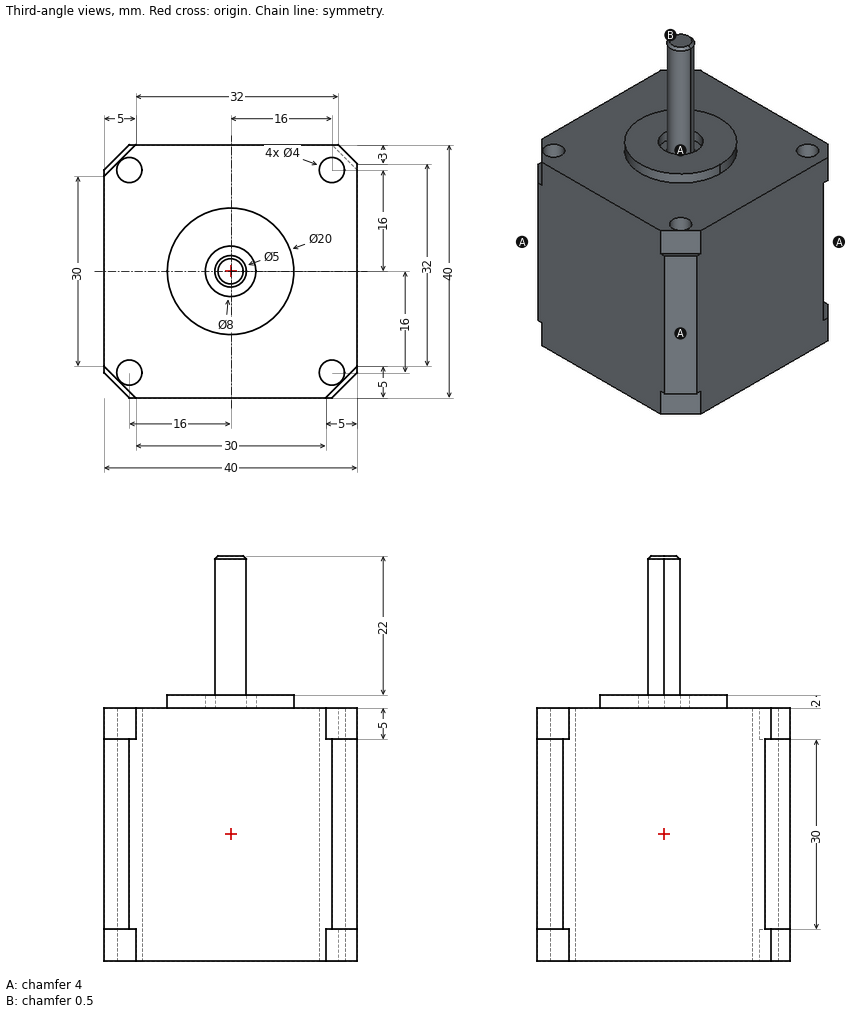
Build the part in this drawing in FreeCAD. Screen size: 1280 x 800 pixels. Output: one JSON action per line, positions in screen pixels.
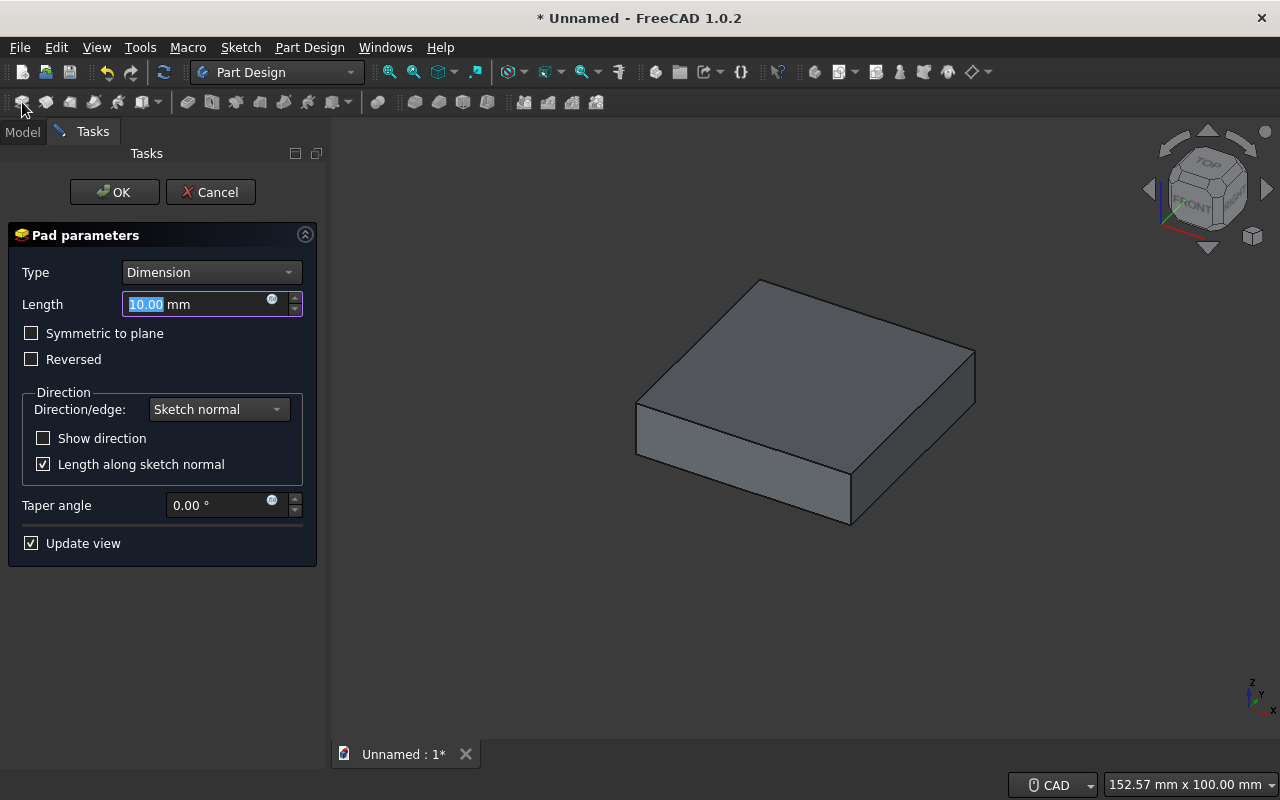
{"action": "type", "text": "30"}
{"action": "key", "text": "Tab"}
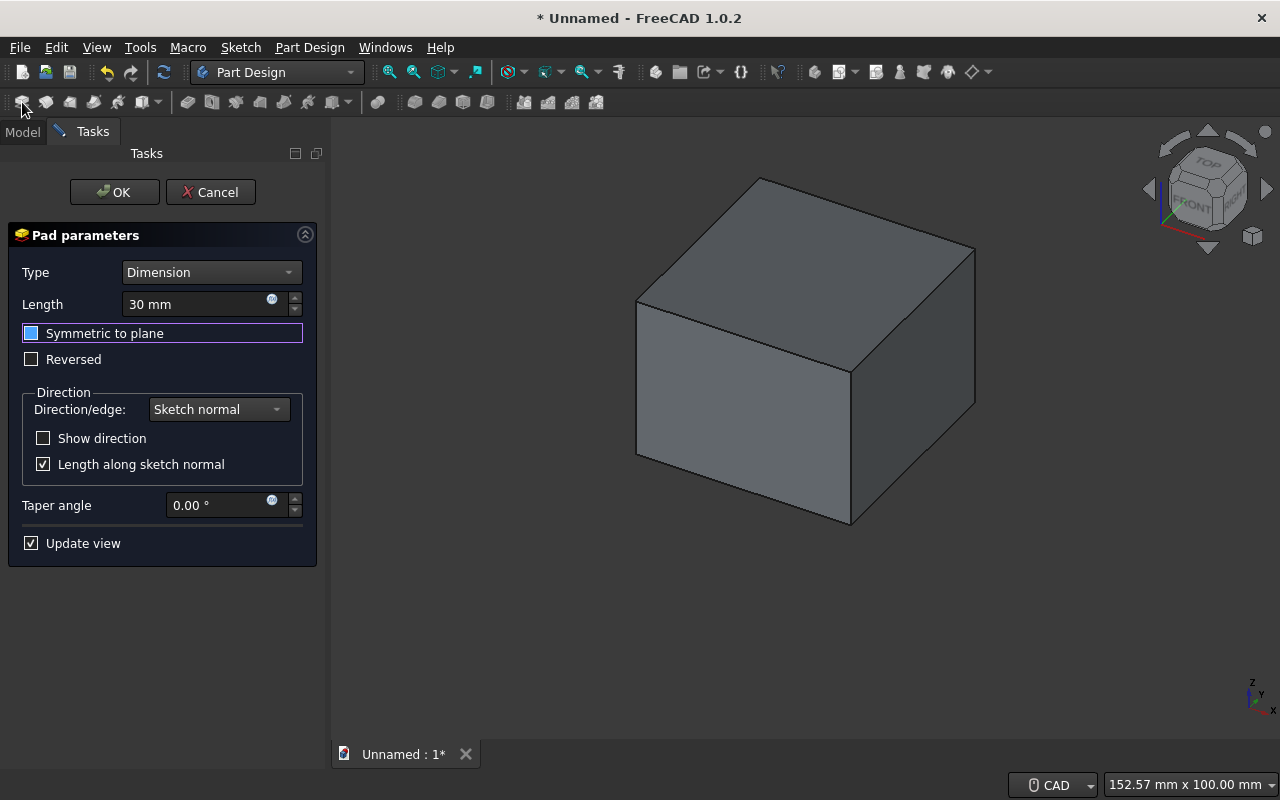
{"action": "left_click", "coordinate": [30, 333]}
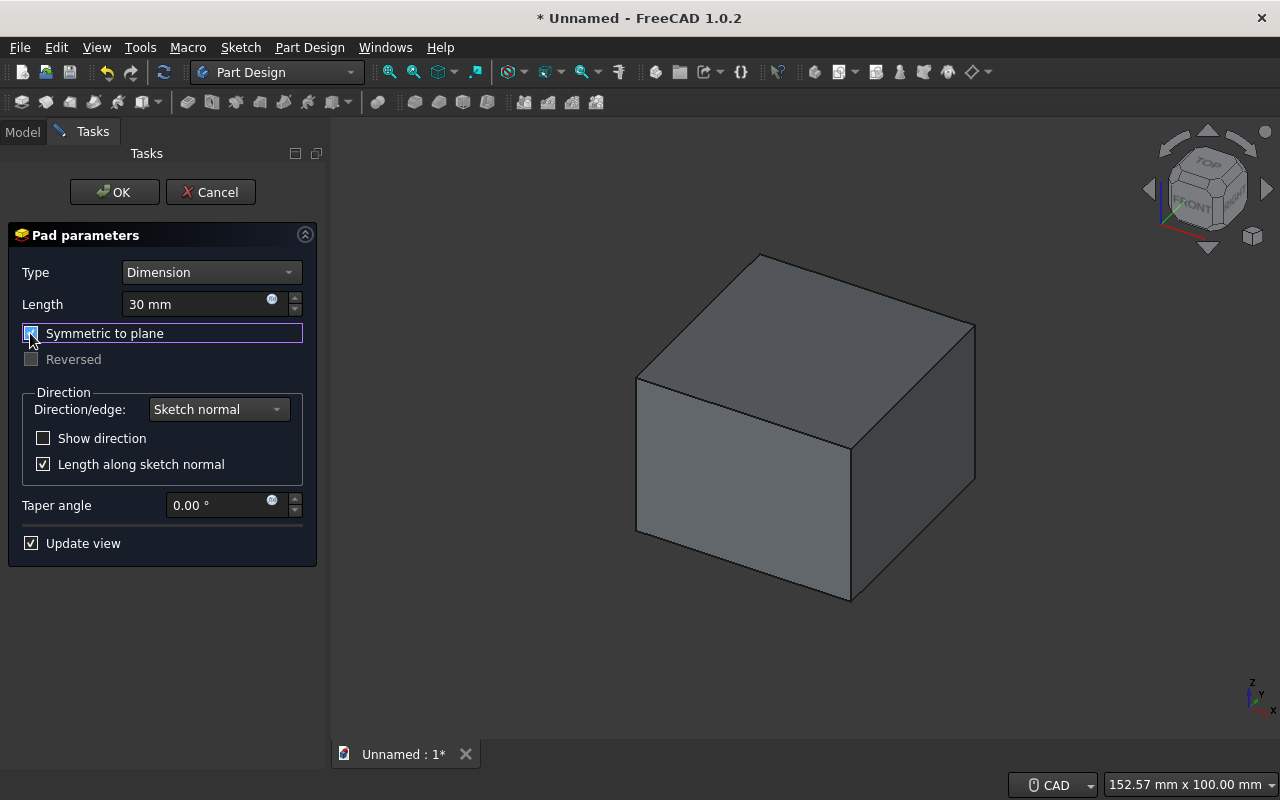
{"action": "left_click", "coordinate": [115, 192]}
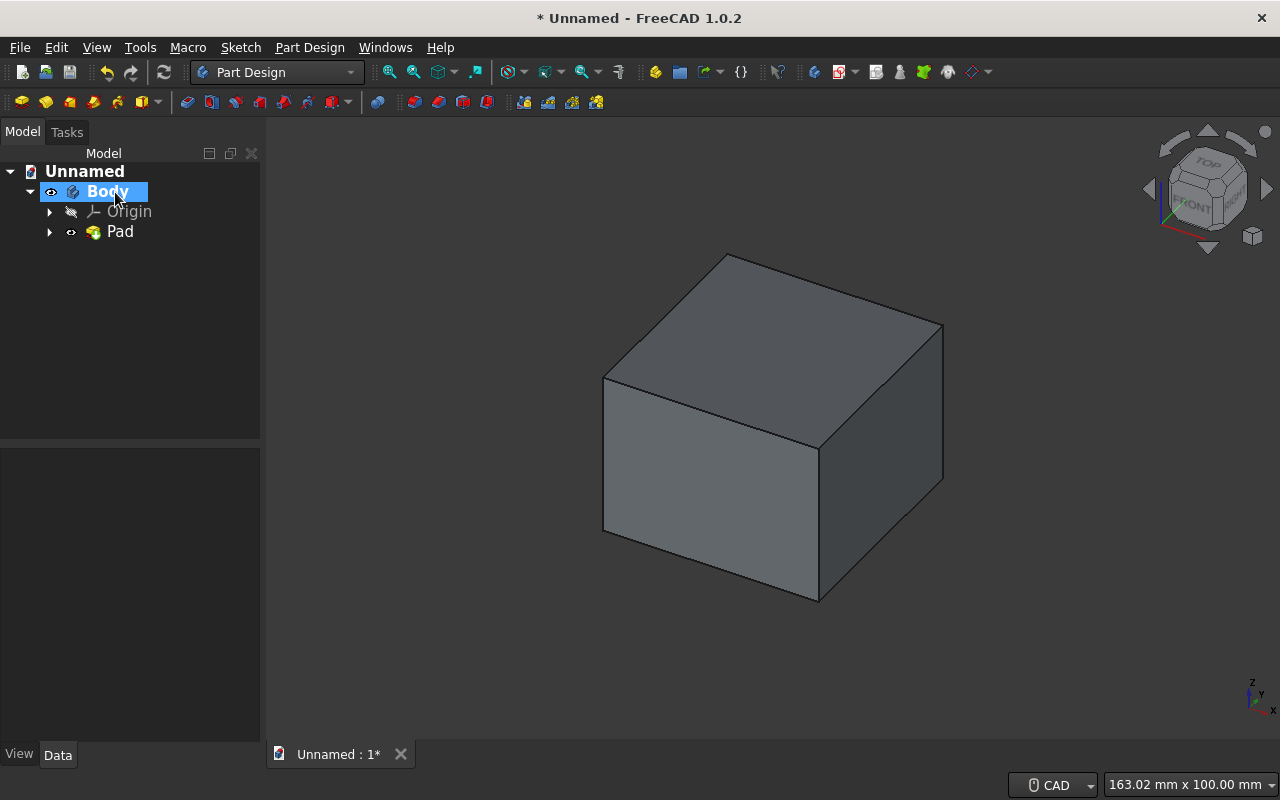
{"action": "left_click", "coordinate": [819, 524]}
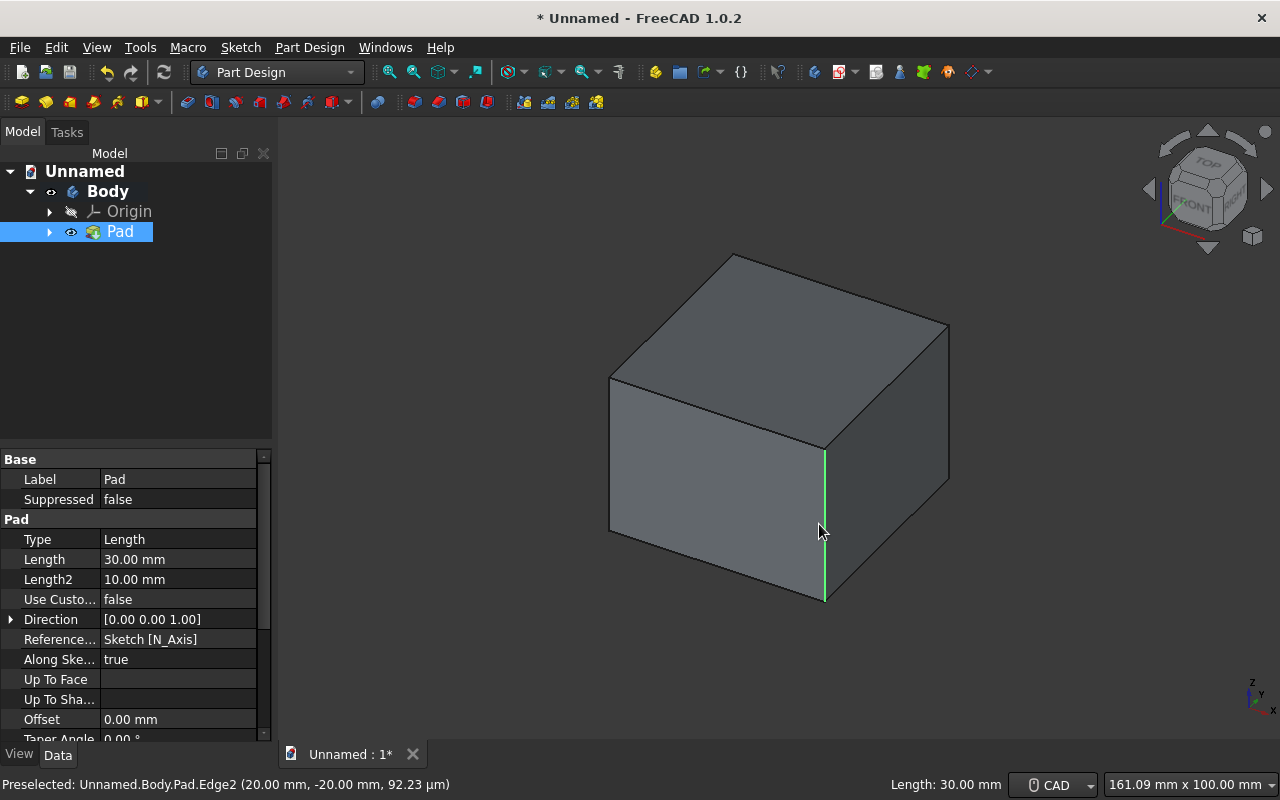
{"action": "key", "text": "0"}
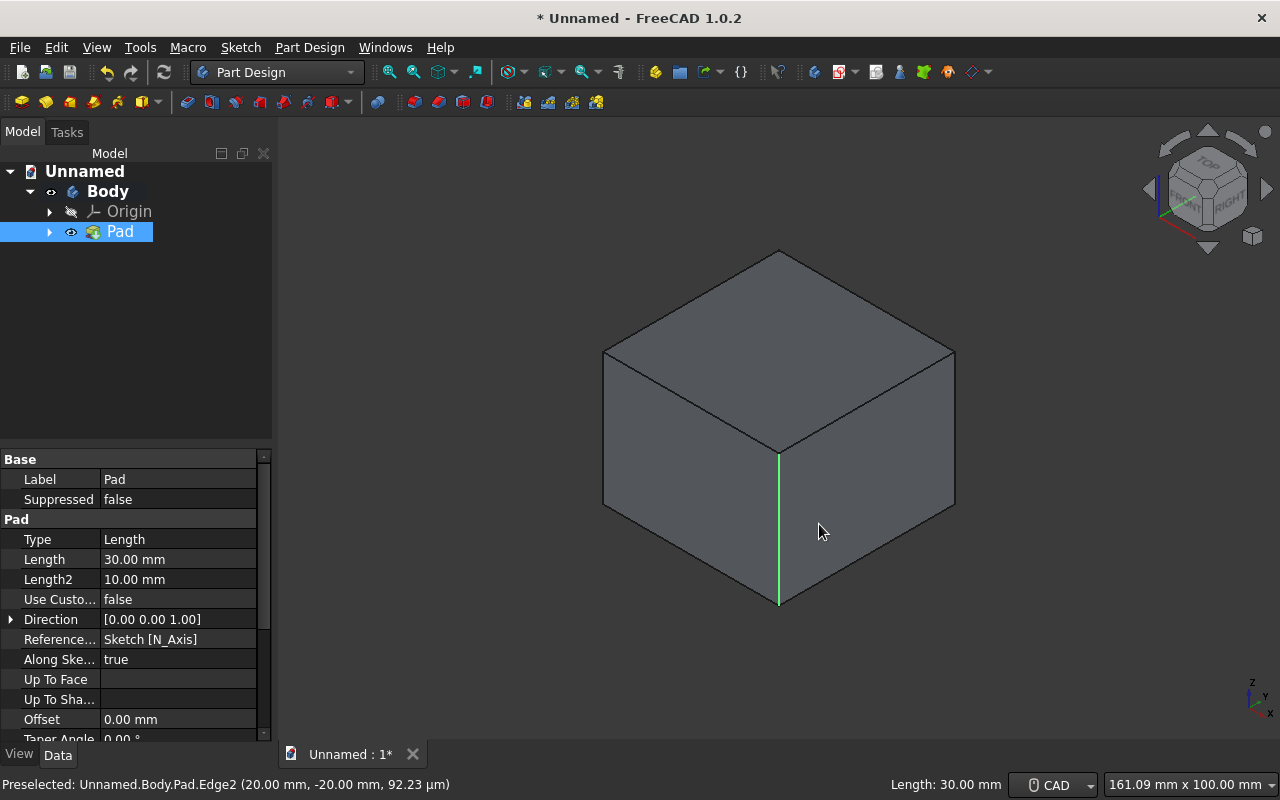
{"action": "key", "text": "2"}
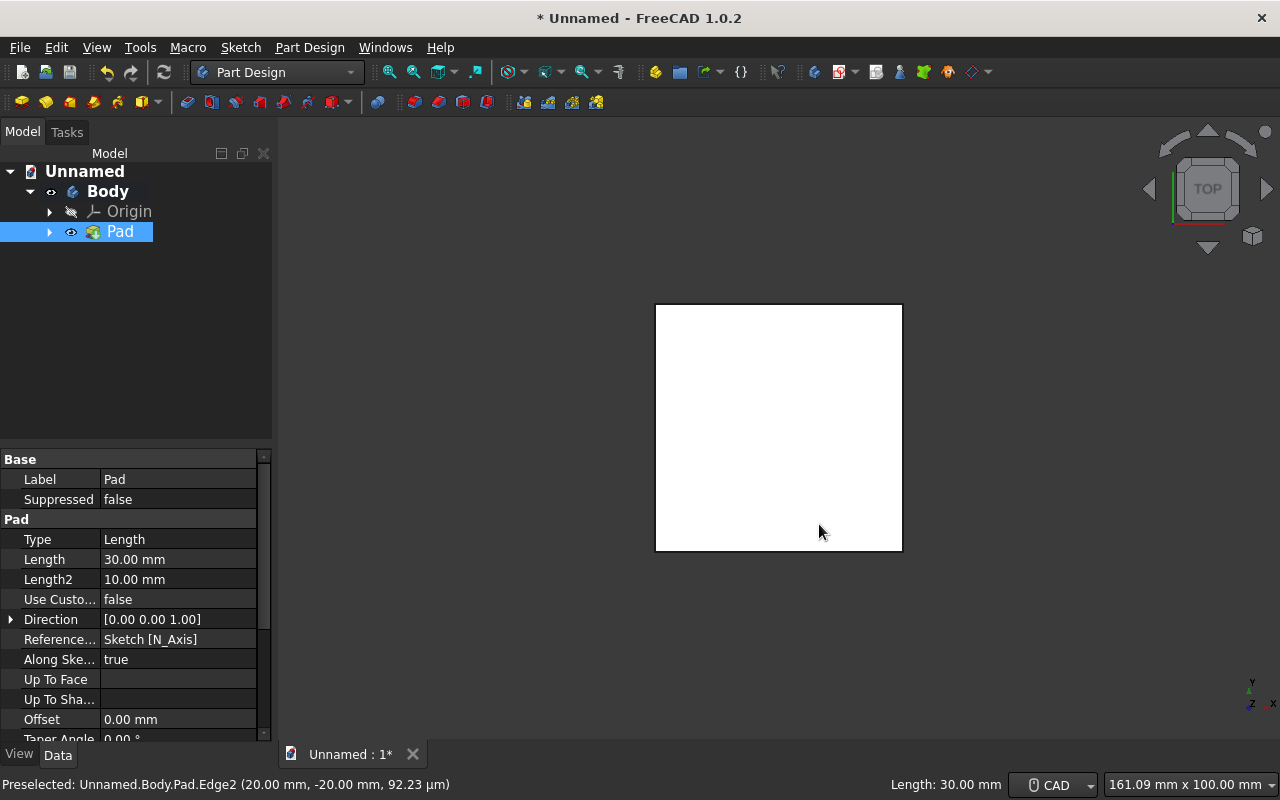
{"action": "left_click", "coordinate": [390, 72]}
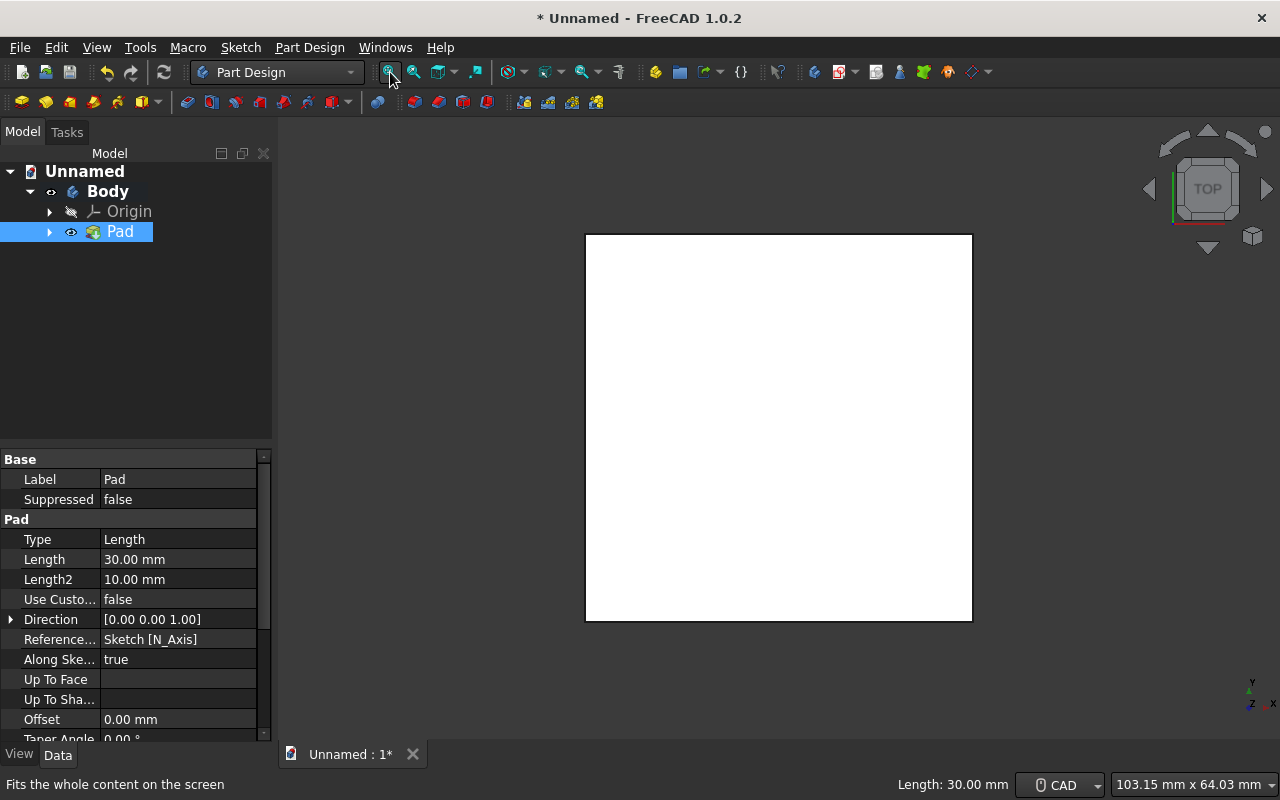
{"action": "key", "text": "1"}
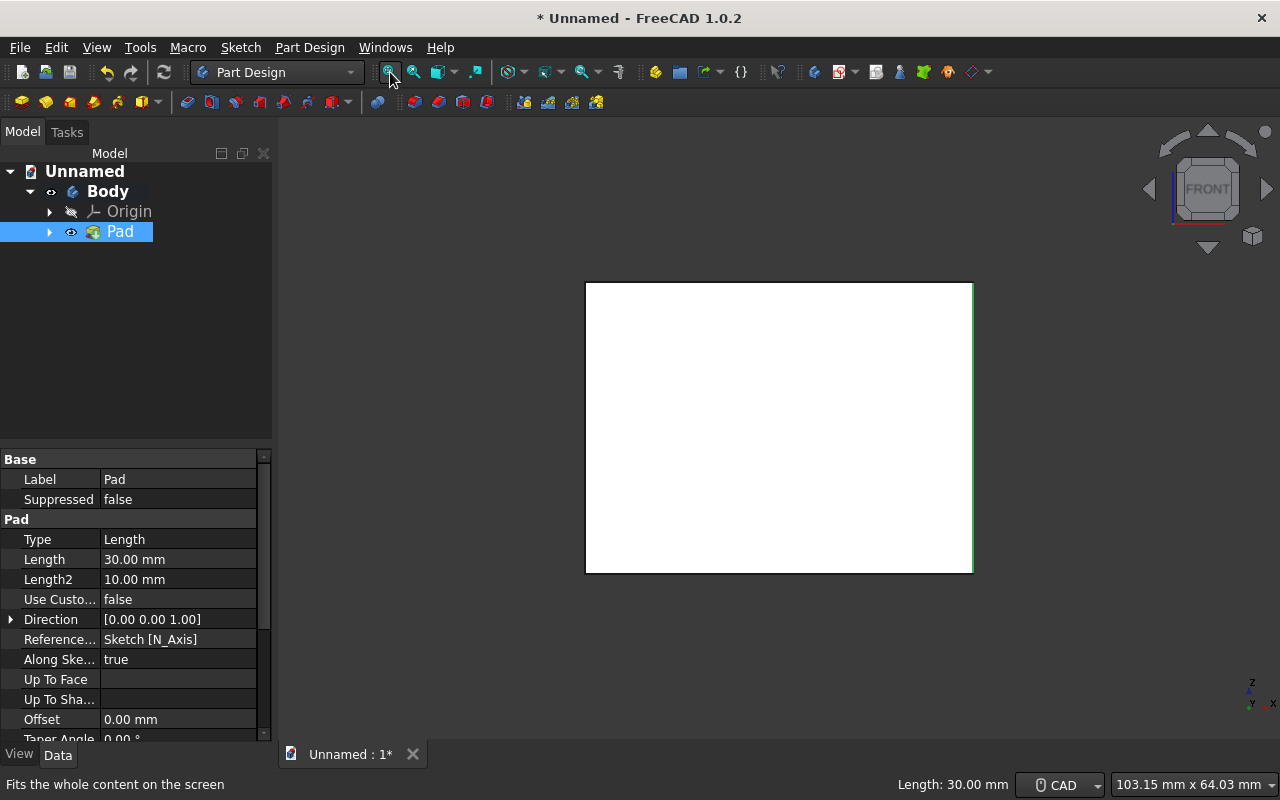
{"action": "left_click", "coordinate": [585, 427], "text": "ctrl"}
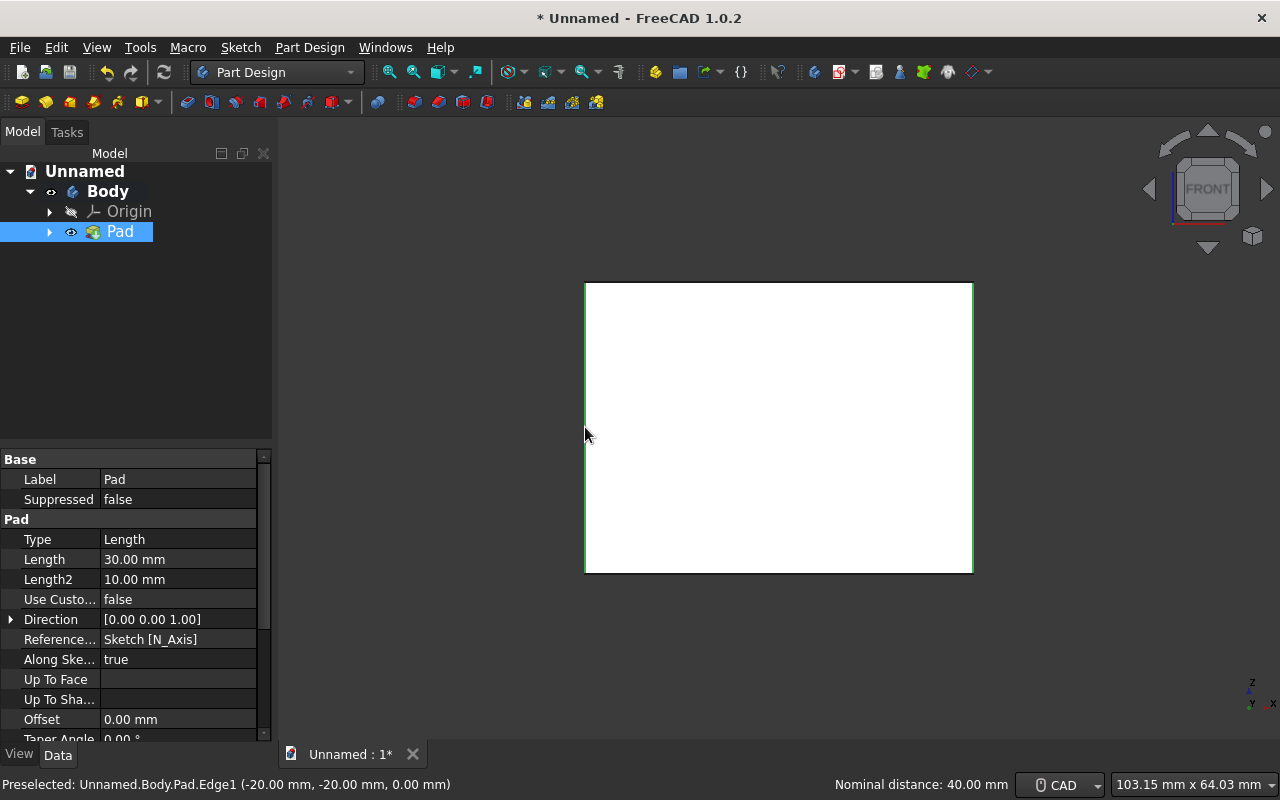
{"action": "key", "text": "3"}